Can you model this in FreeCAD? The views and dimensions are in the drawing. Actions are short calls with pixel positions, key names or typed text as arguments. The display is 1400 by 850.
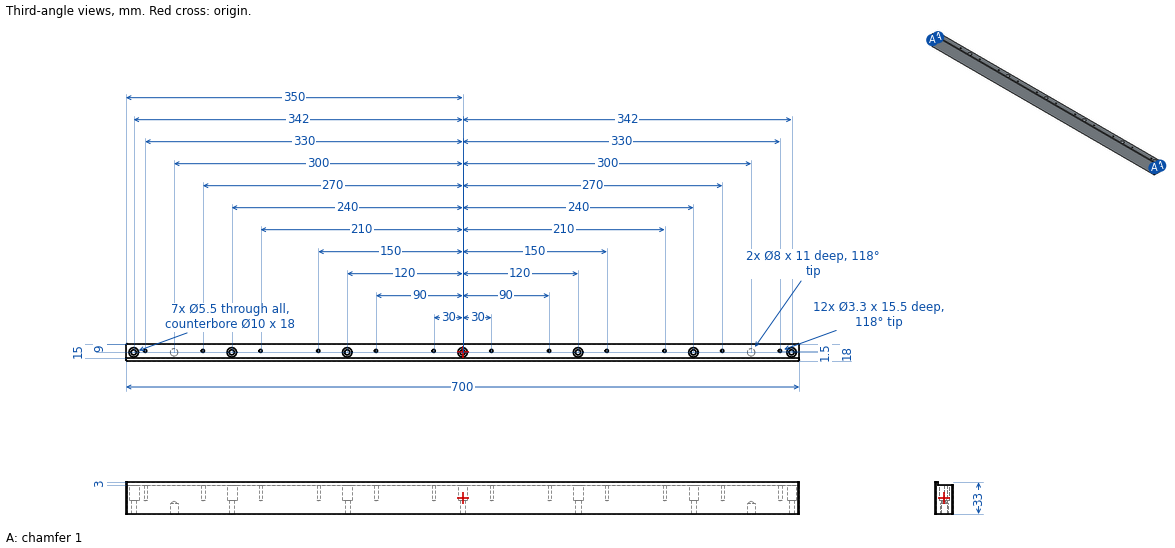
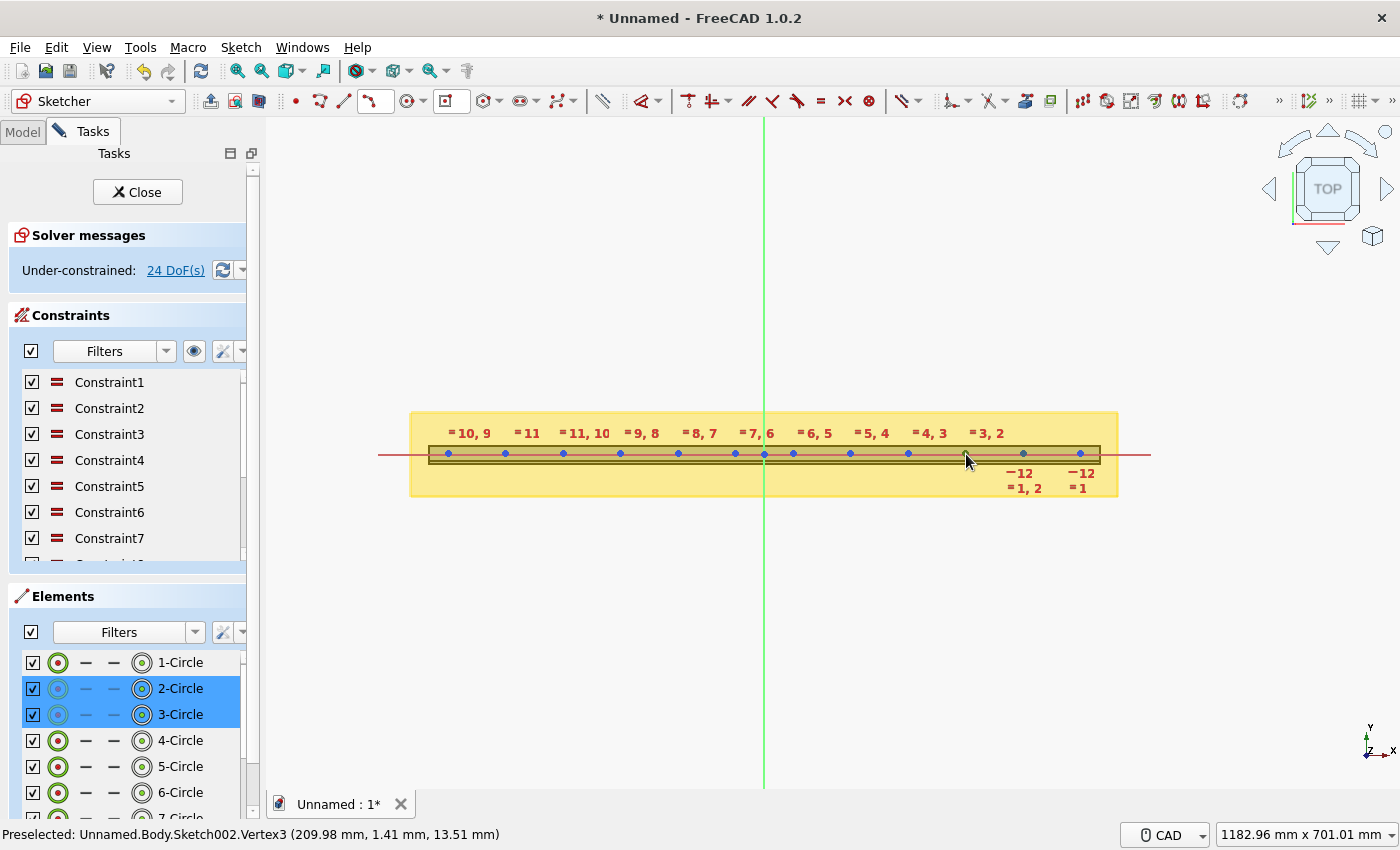
click(730, 102)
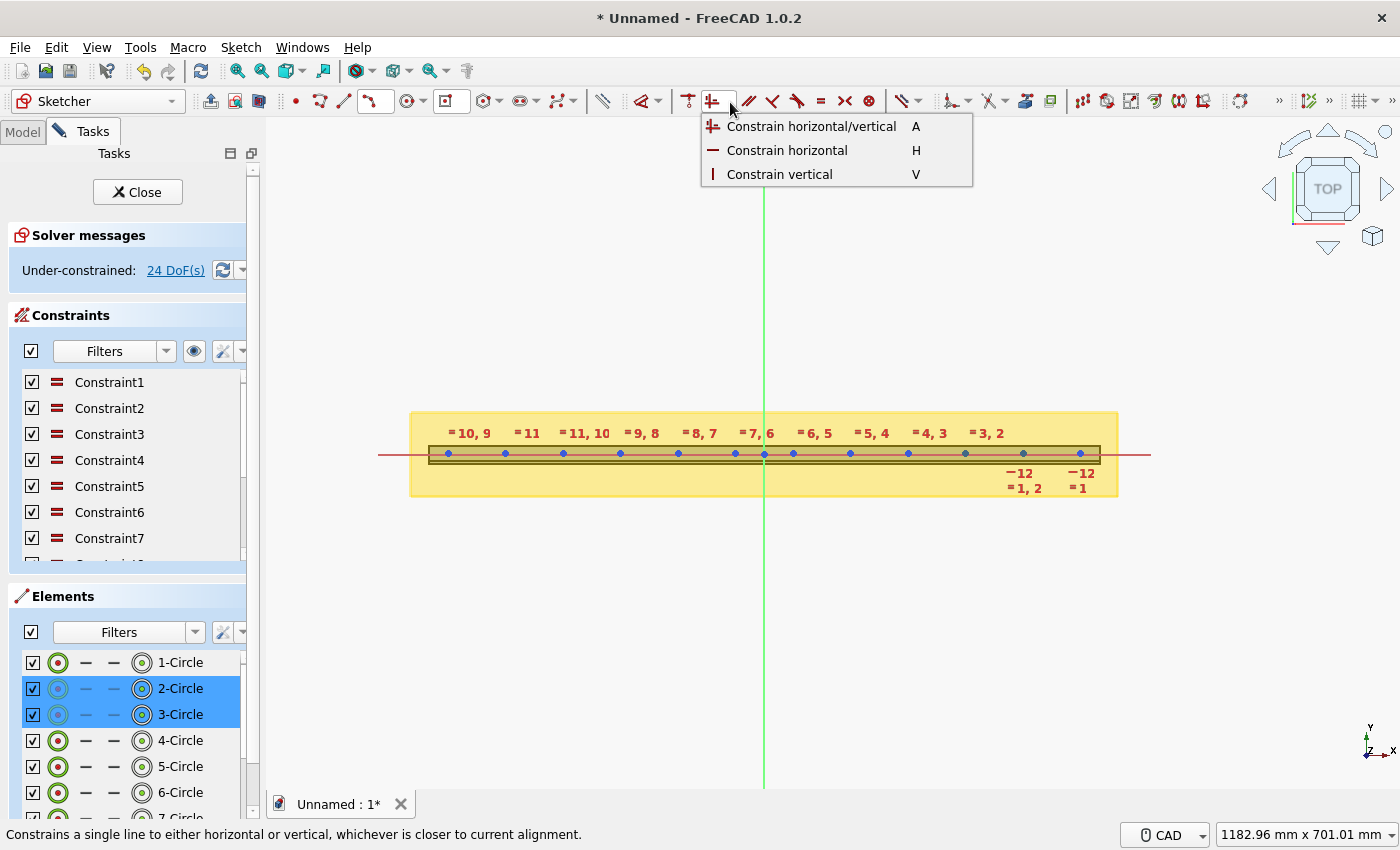
click(837, 150)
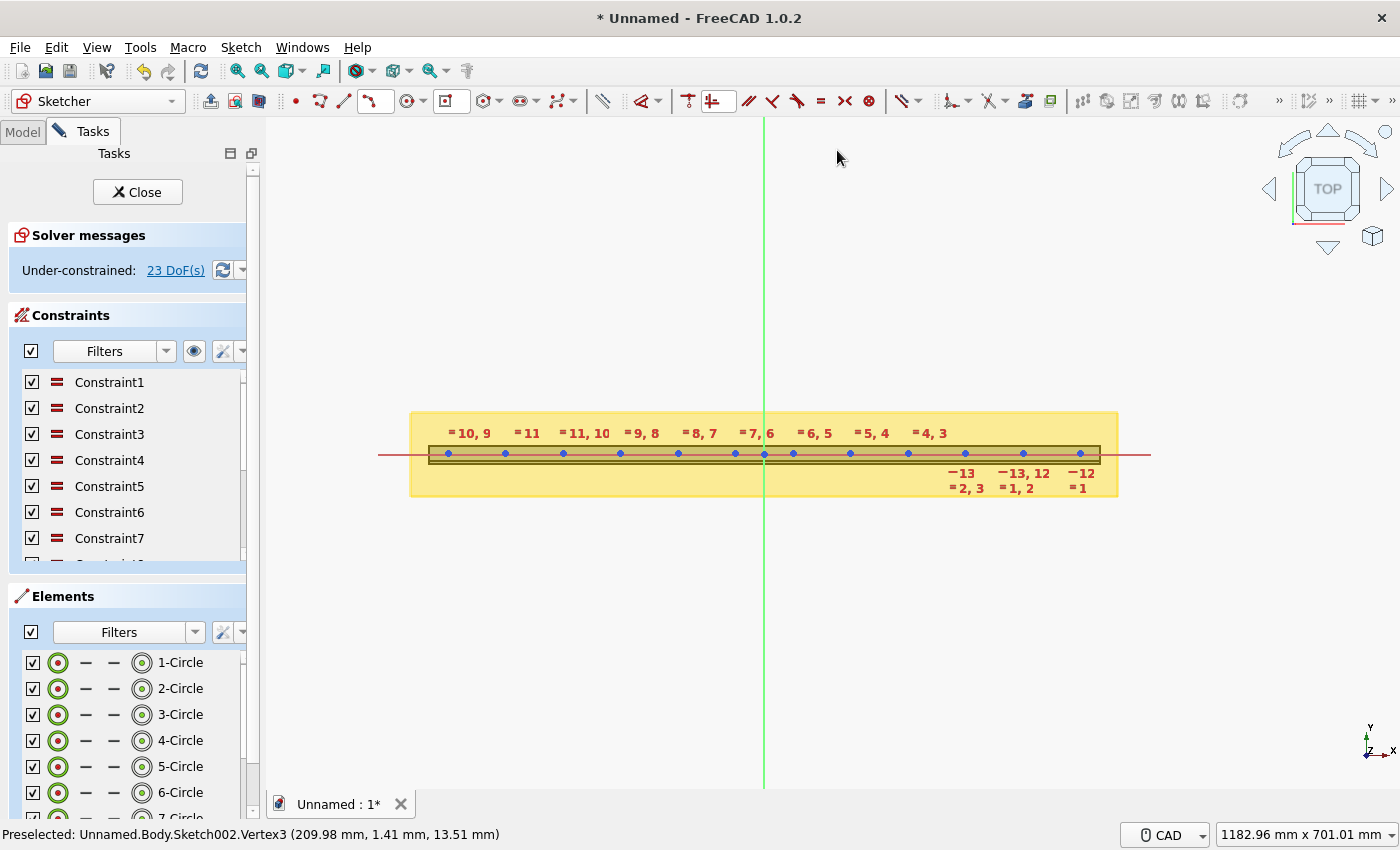
click(966, 453)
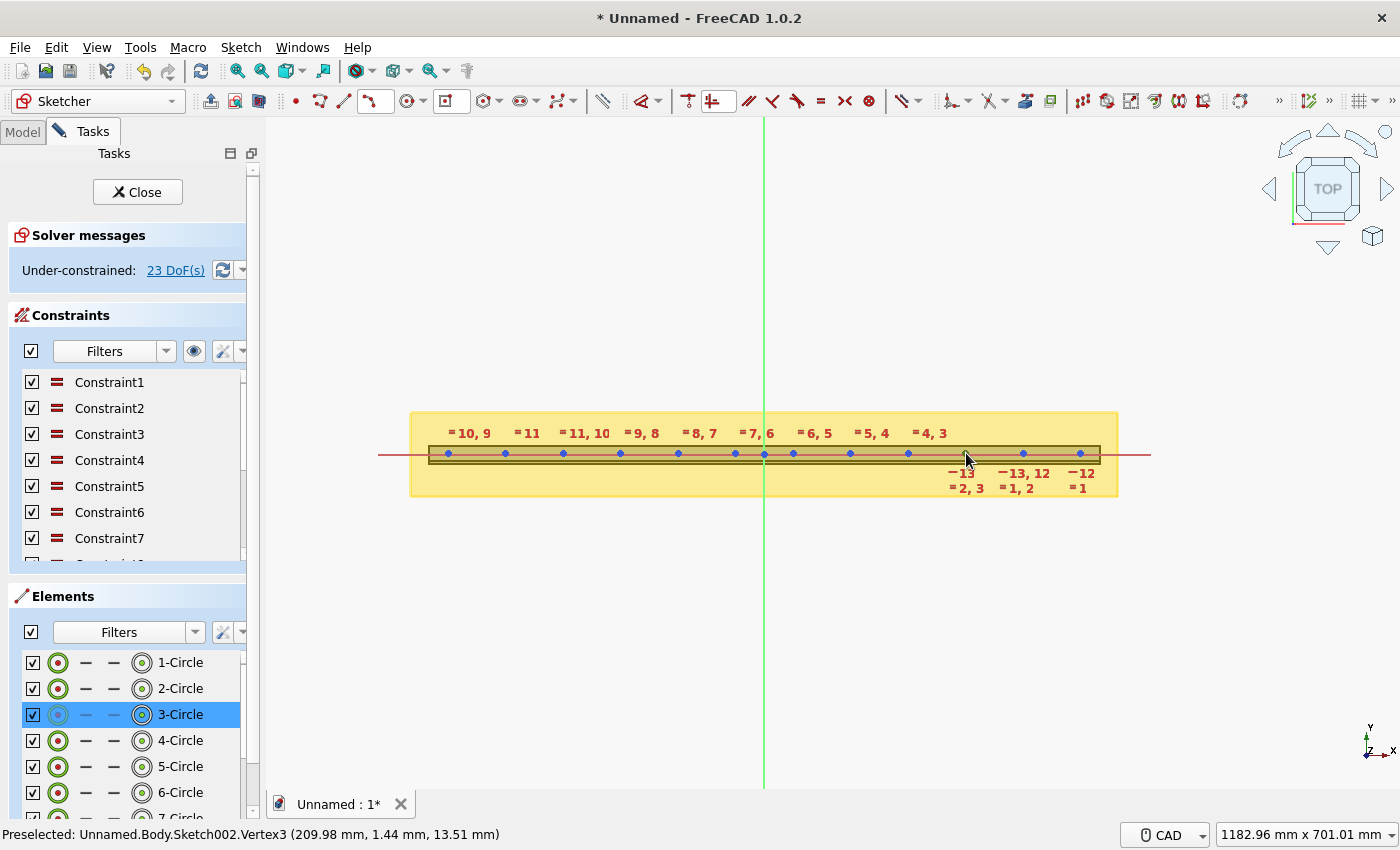
click(908, 454)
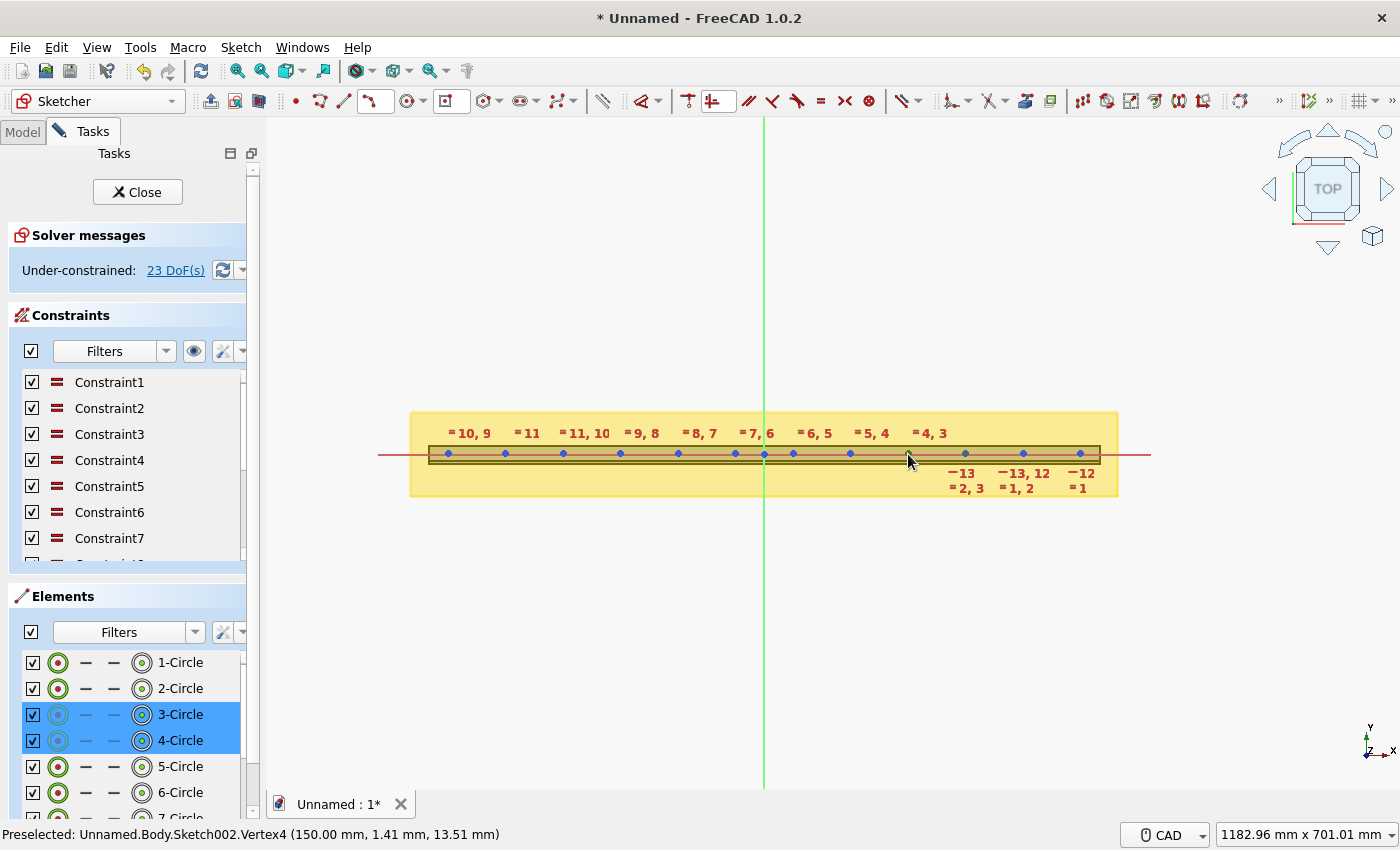
key(h)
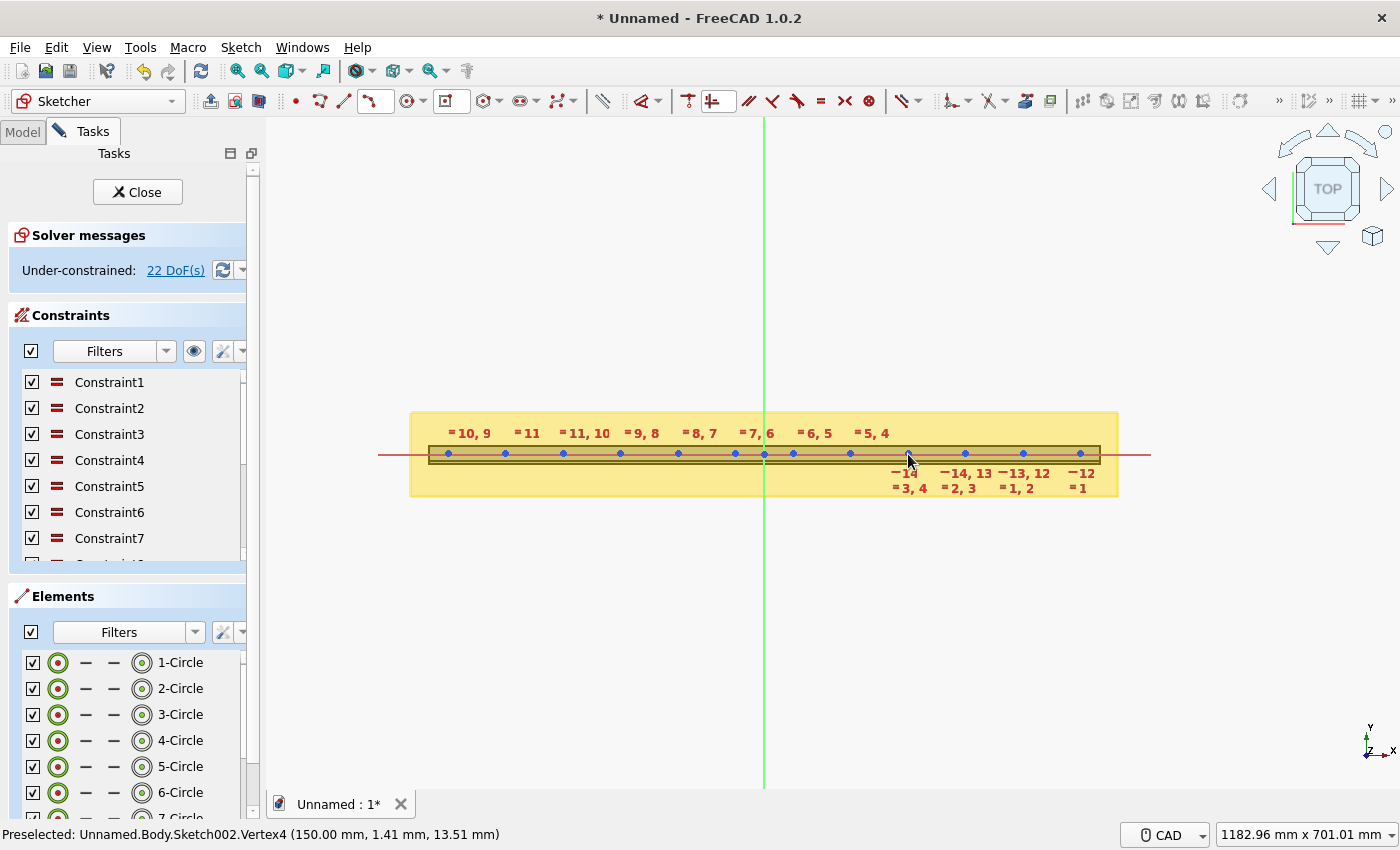
click(908, 453)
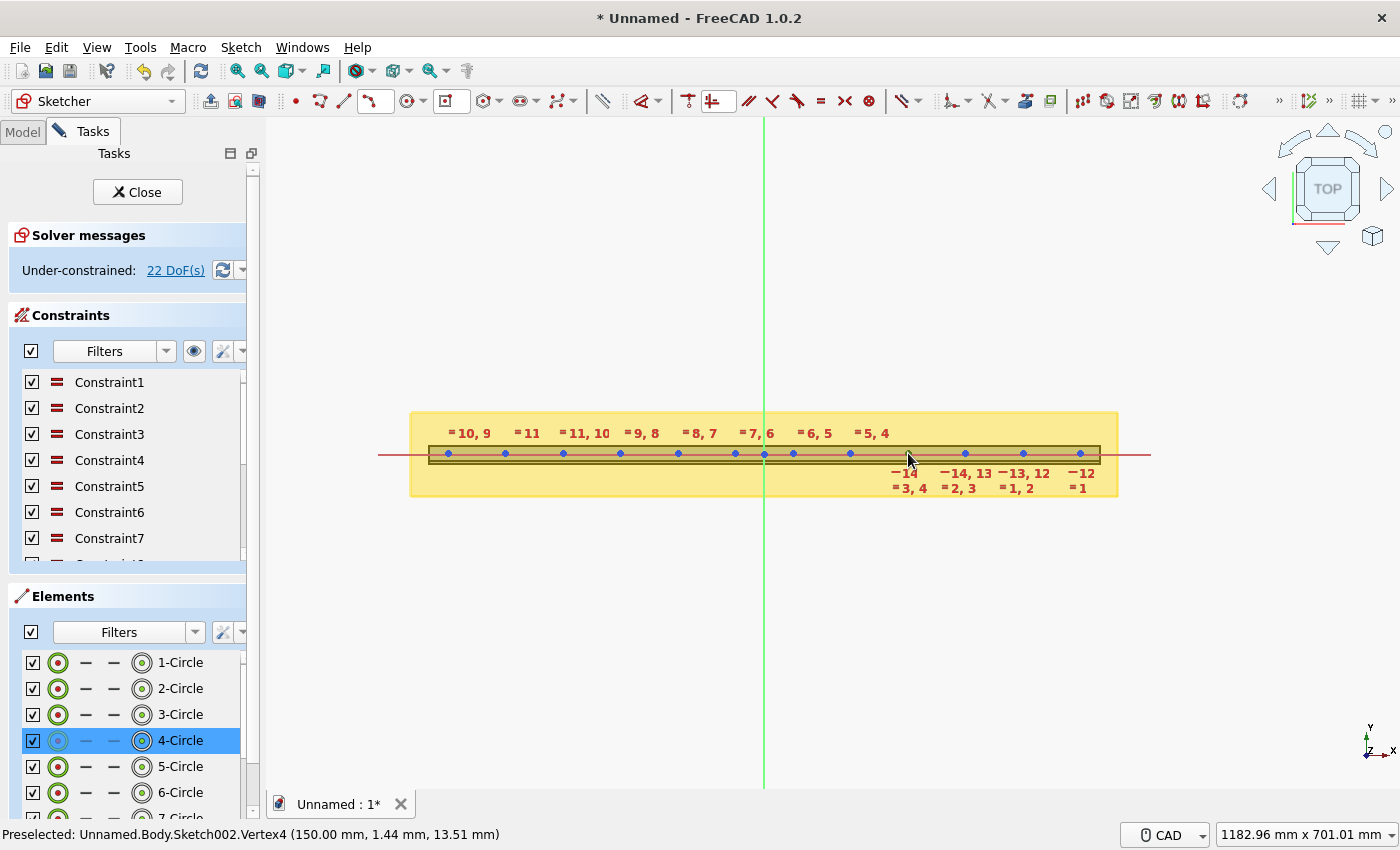
click(851, 454)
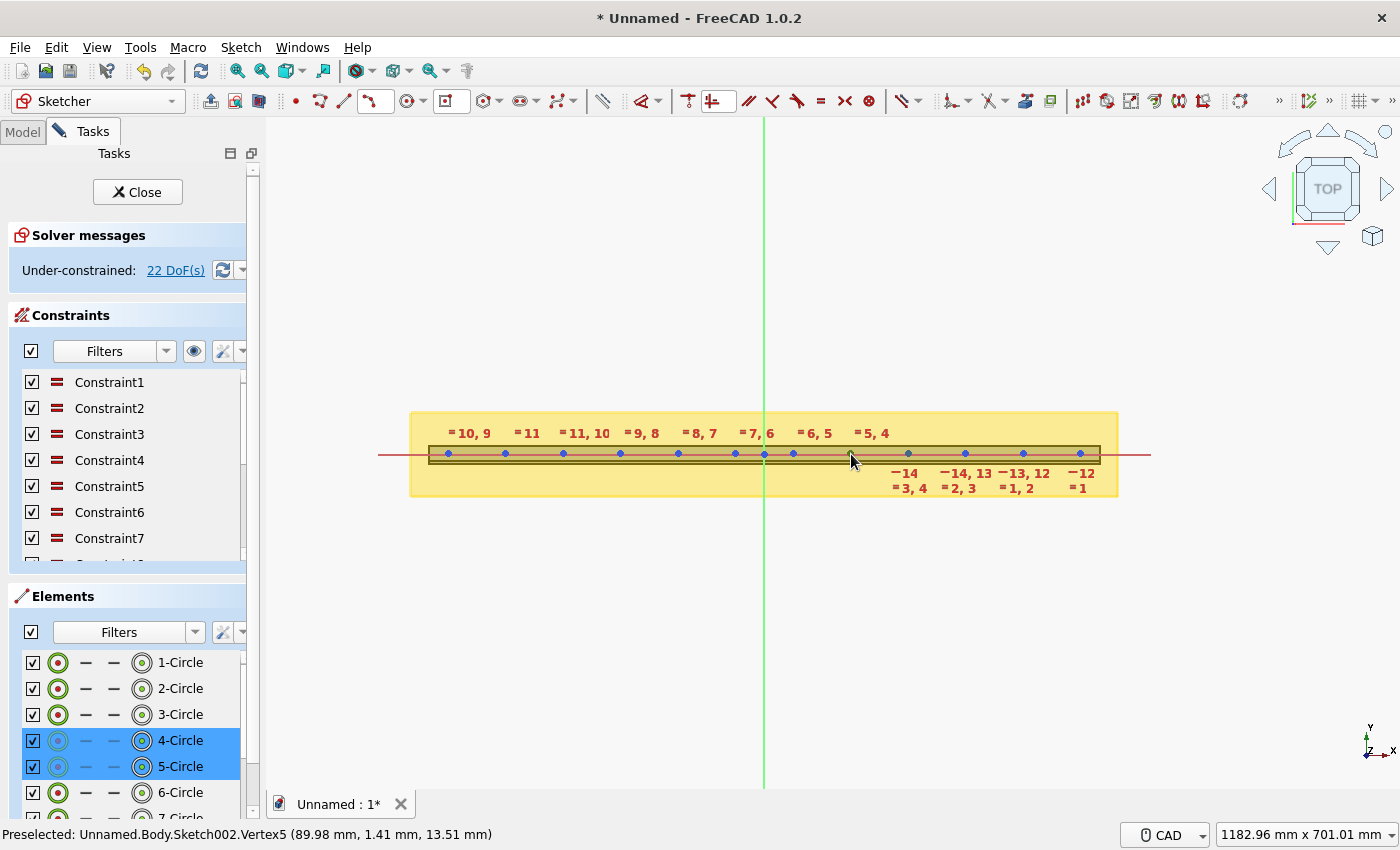
click(730, 102)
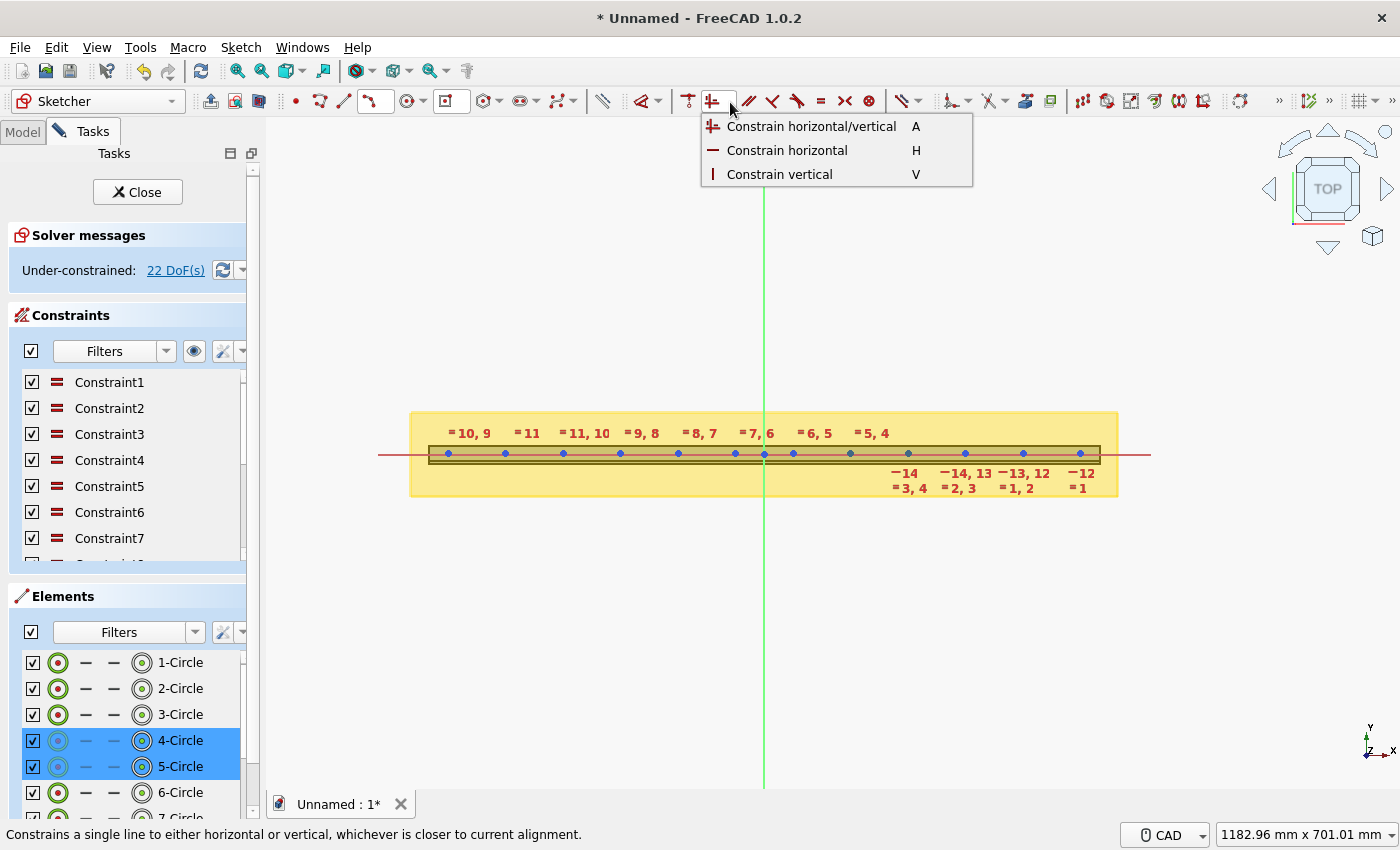
click(837, 150)